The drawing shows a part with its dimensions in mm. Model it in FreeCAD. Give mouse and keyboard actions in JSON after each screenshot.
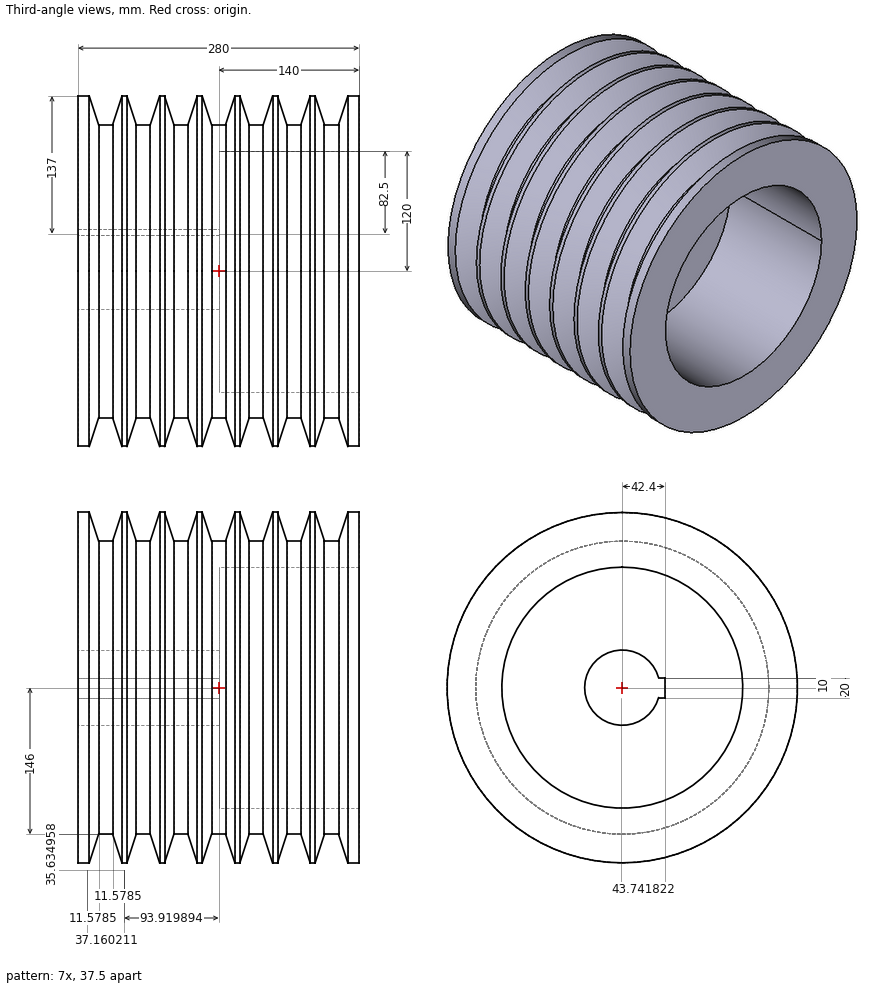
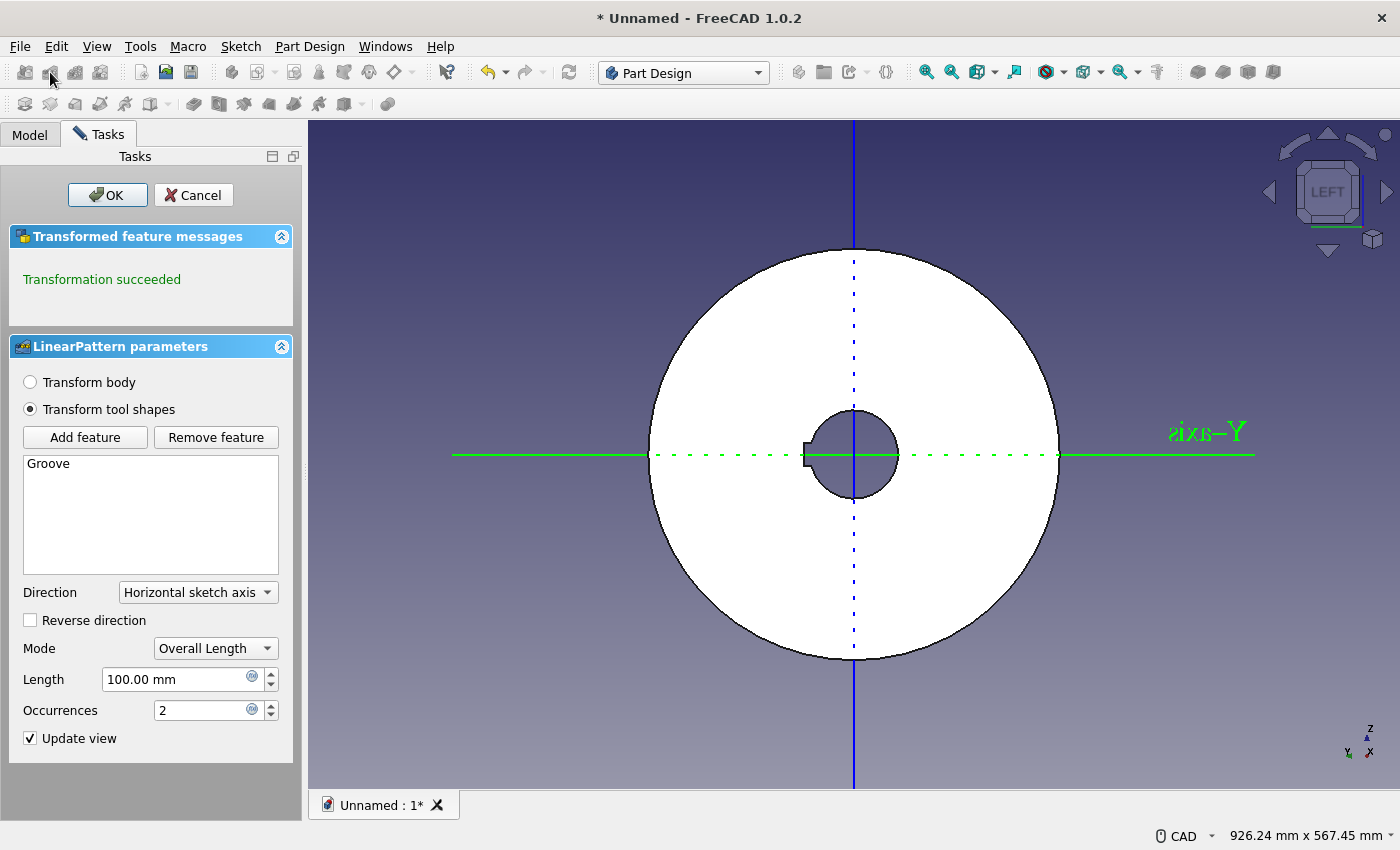
{"action": "left_click", "coordinate": [199, 592]}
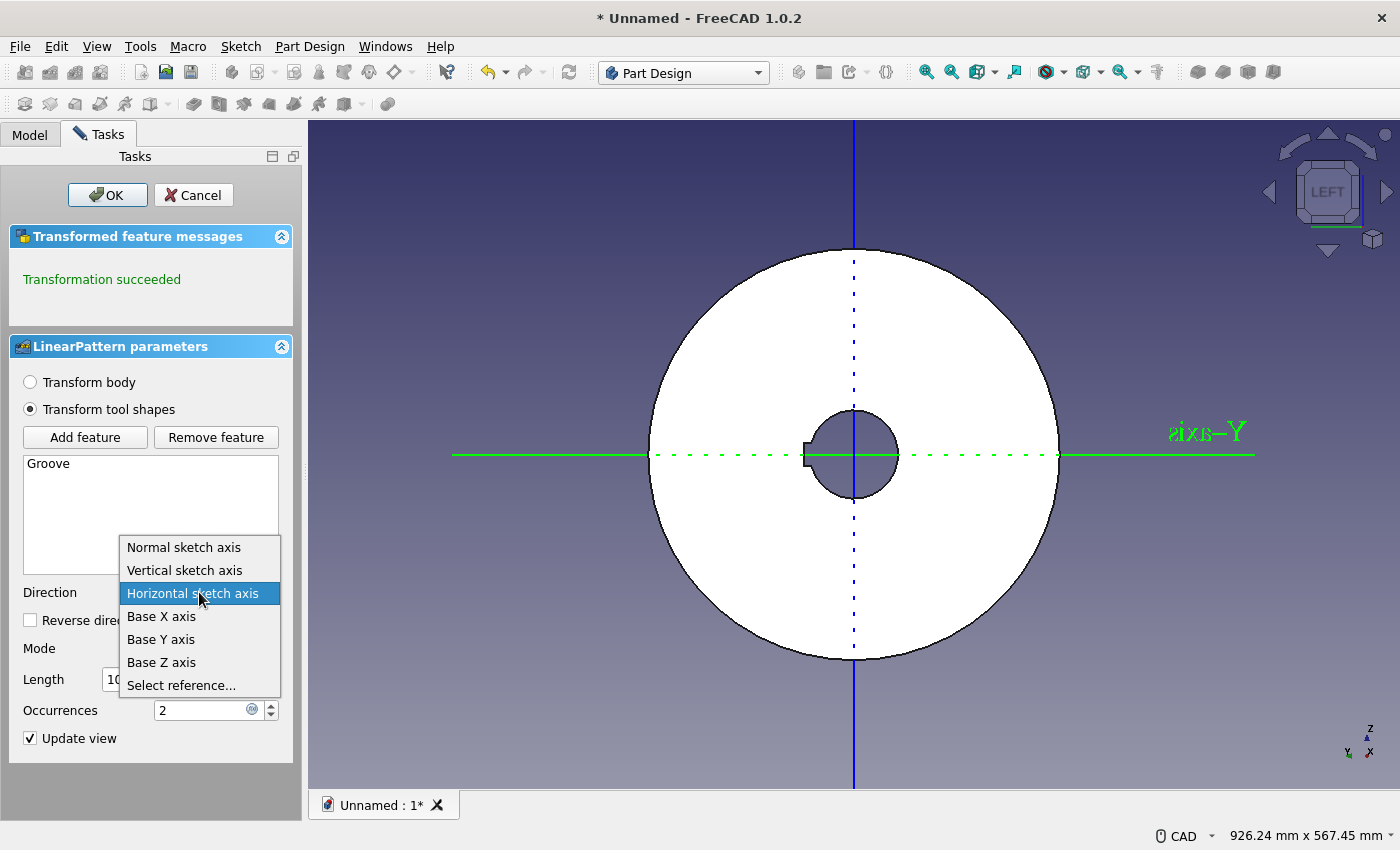
{"action": "left_click", "coordinate": [198, 616]}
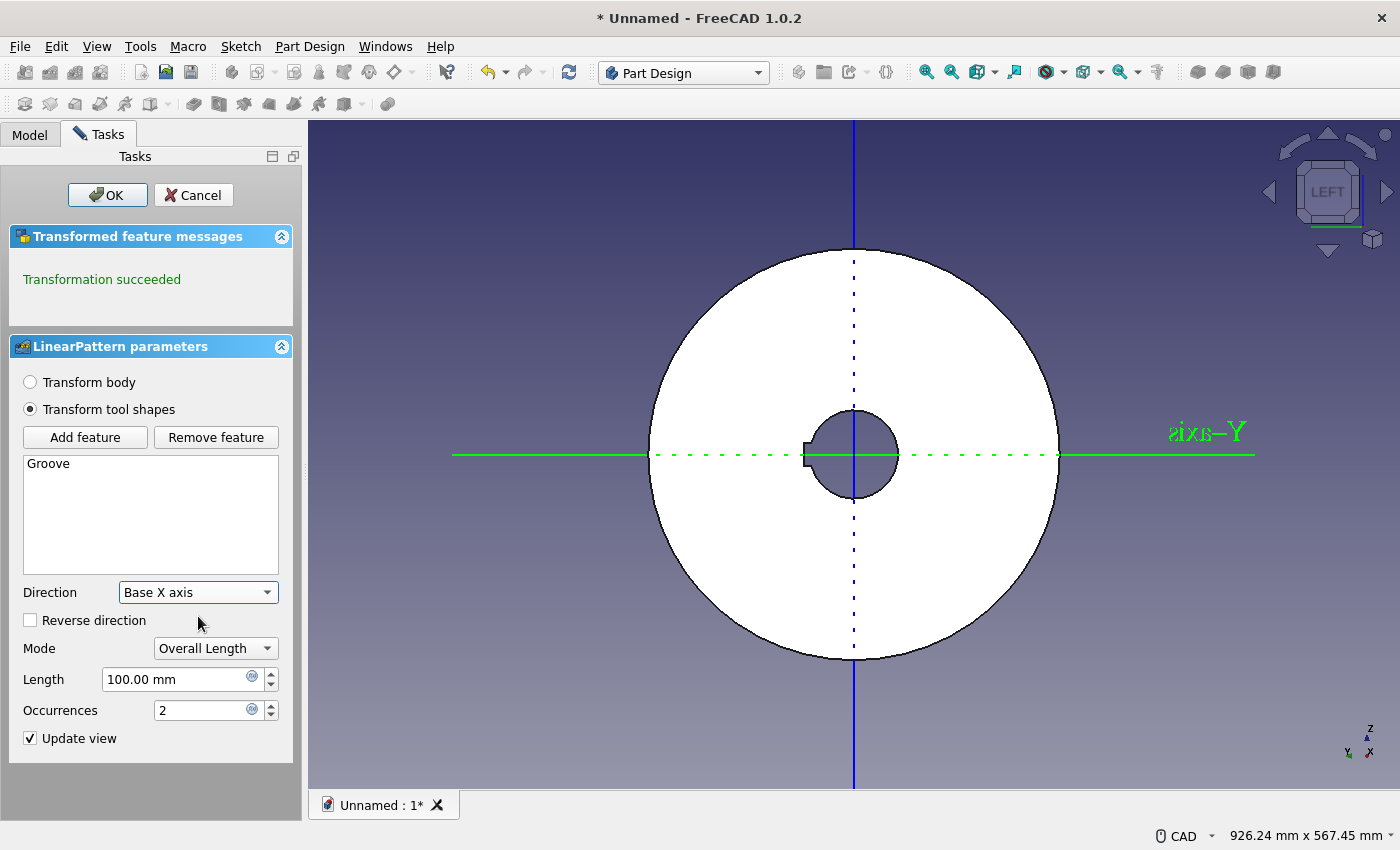
{"action": "left_click", "coordinate": [216, 648]}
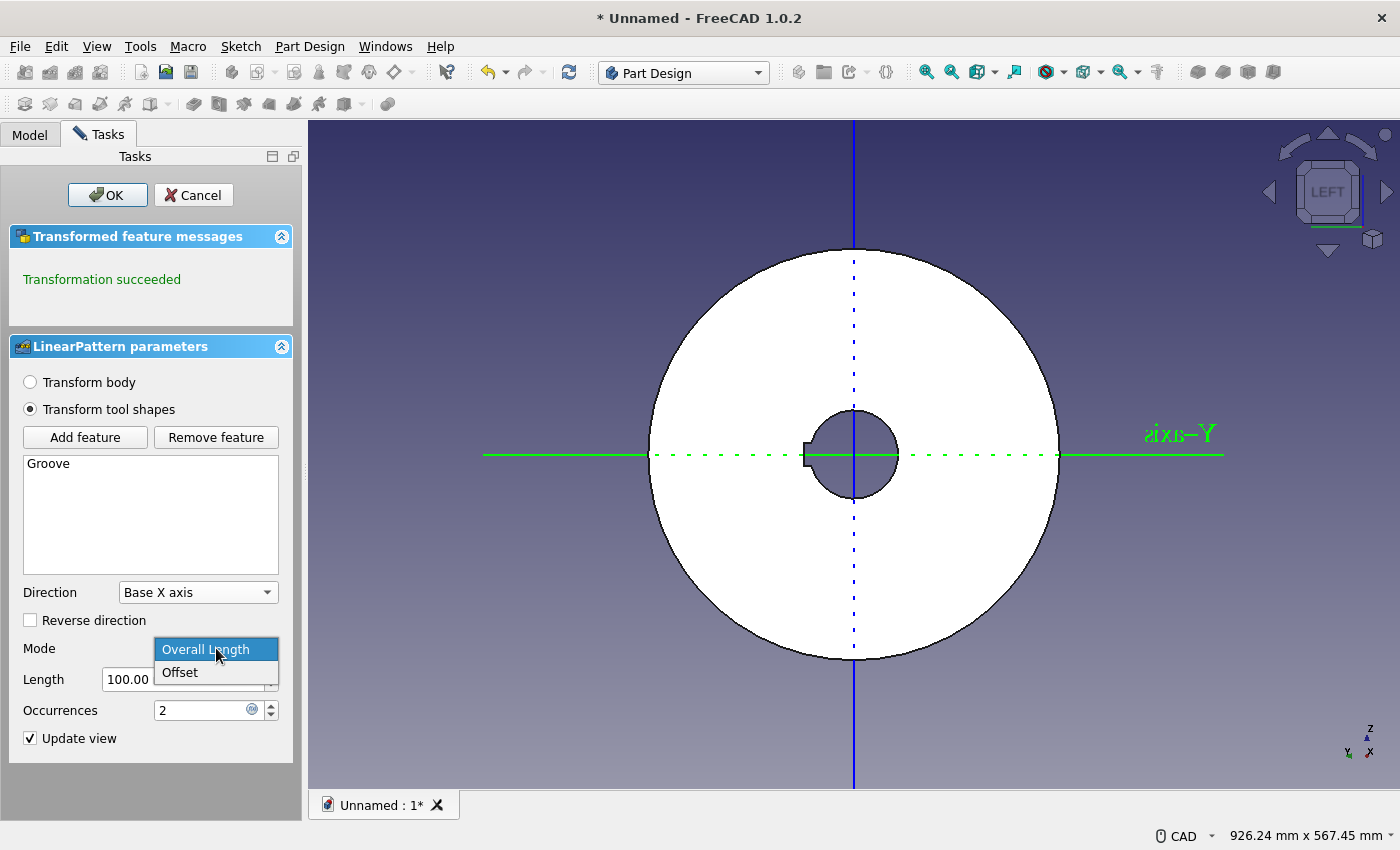
{"action": "left_click", "coordinate": [214, 672]}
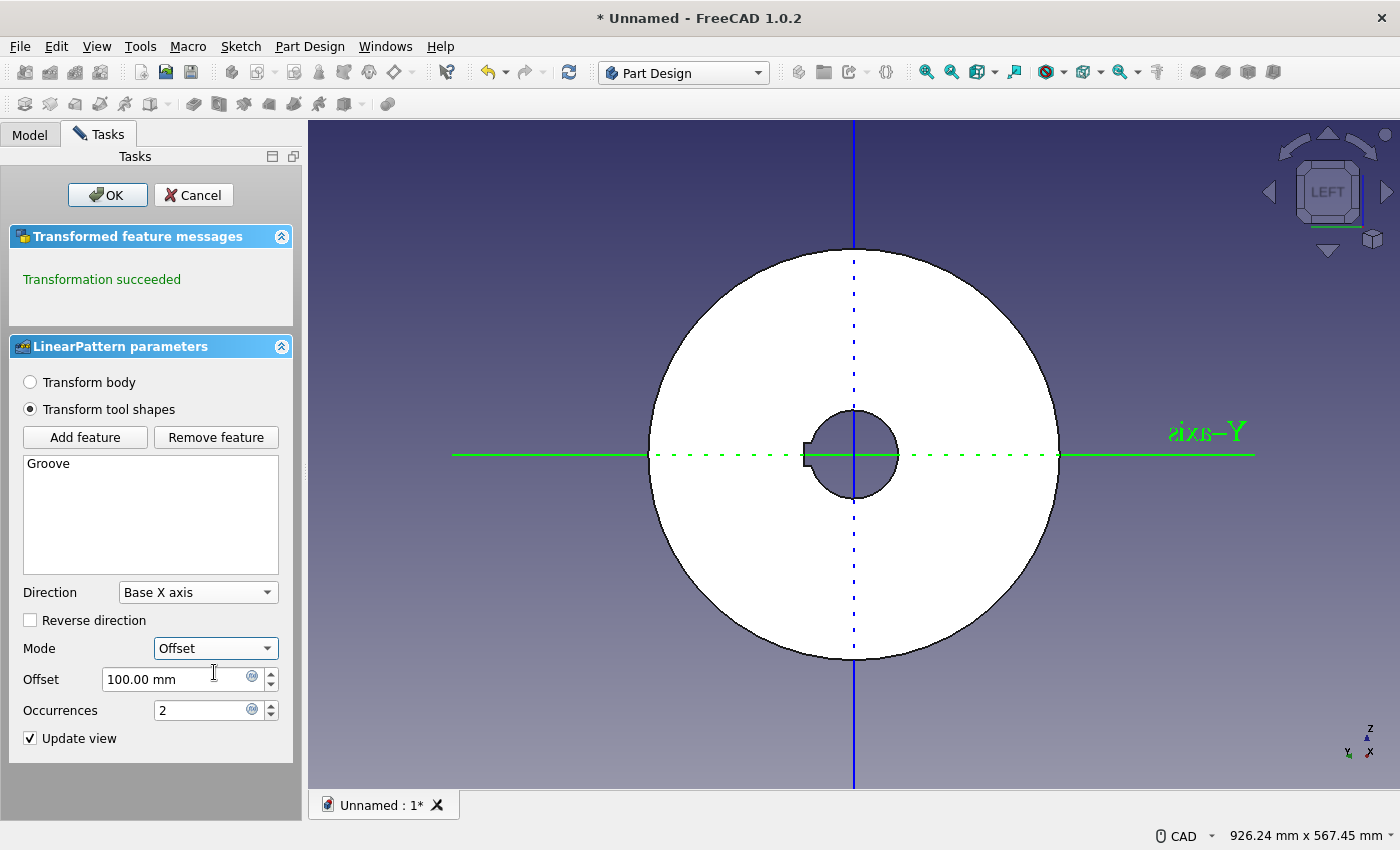
{"action": "triple_click", "coordinate": [184, 680]}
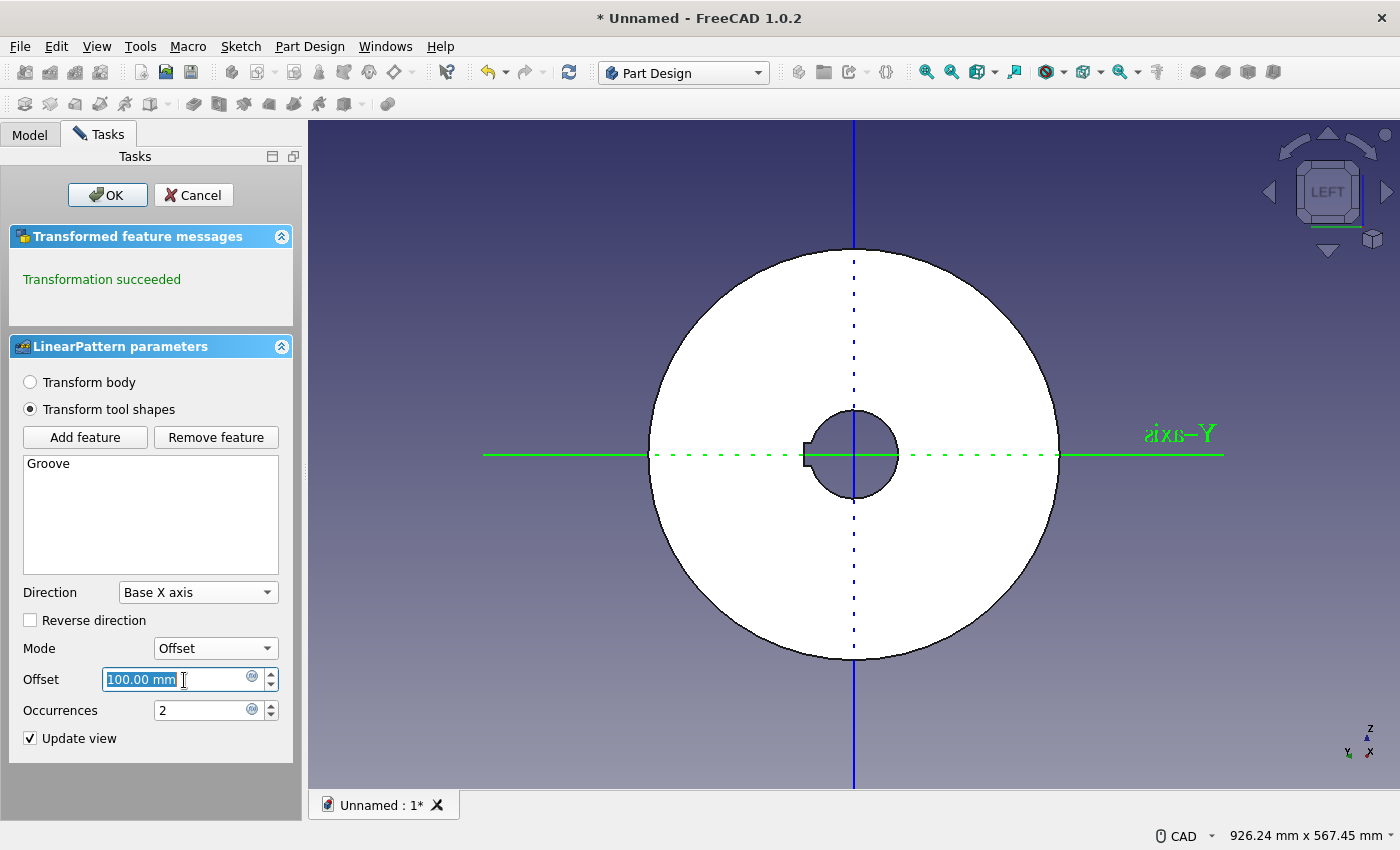
{"action": "type", "text": "37.5"}
{"action": "key", "text": "Tab"}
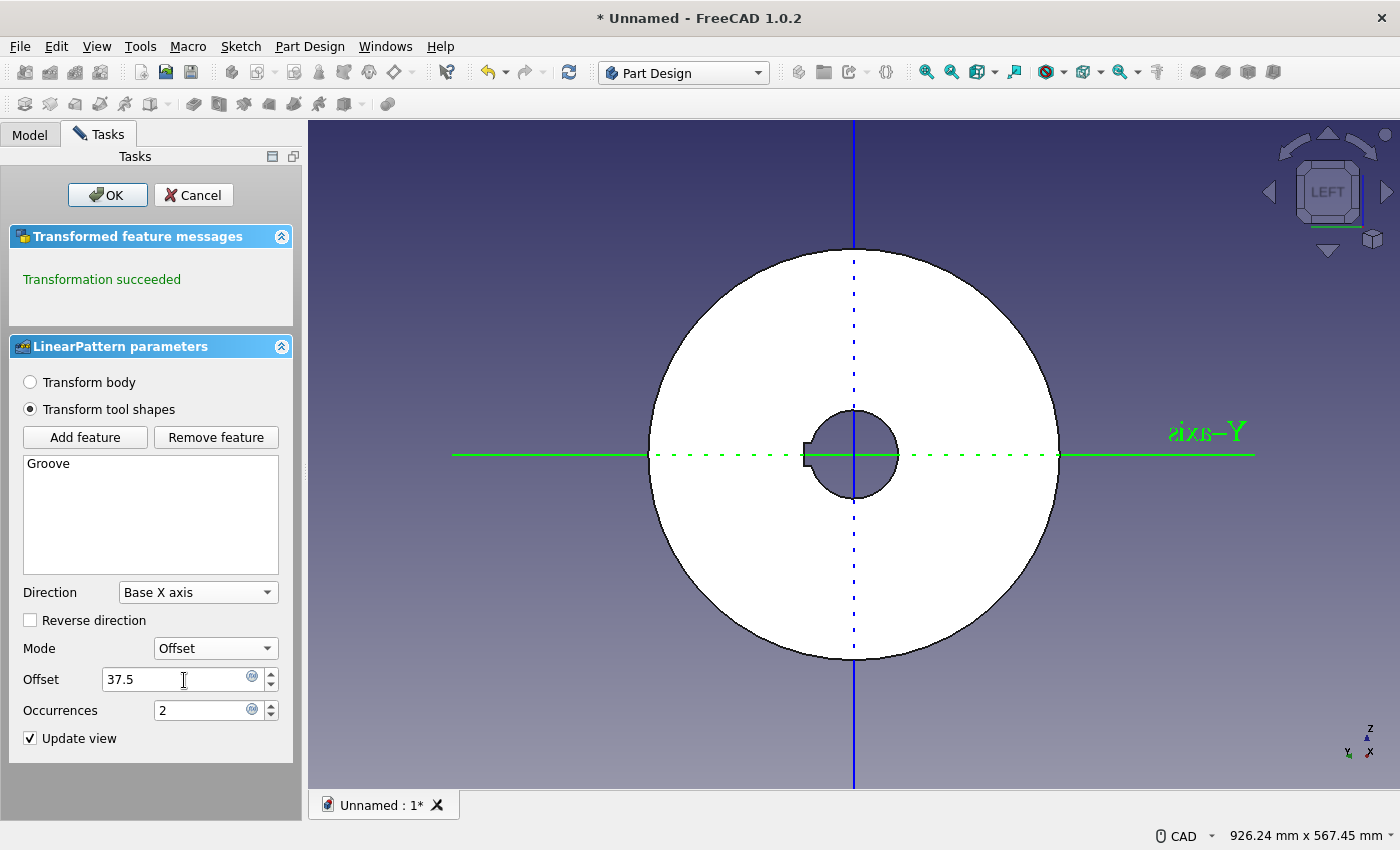
{"action": "triple_click", "coordinate": [210, 710]}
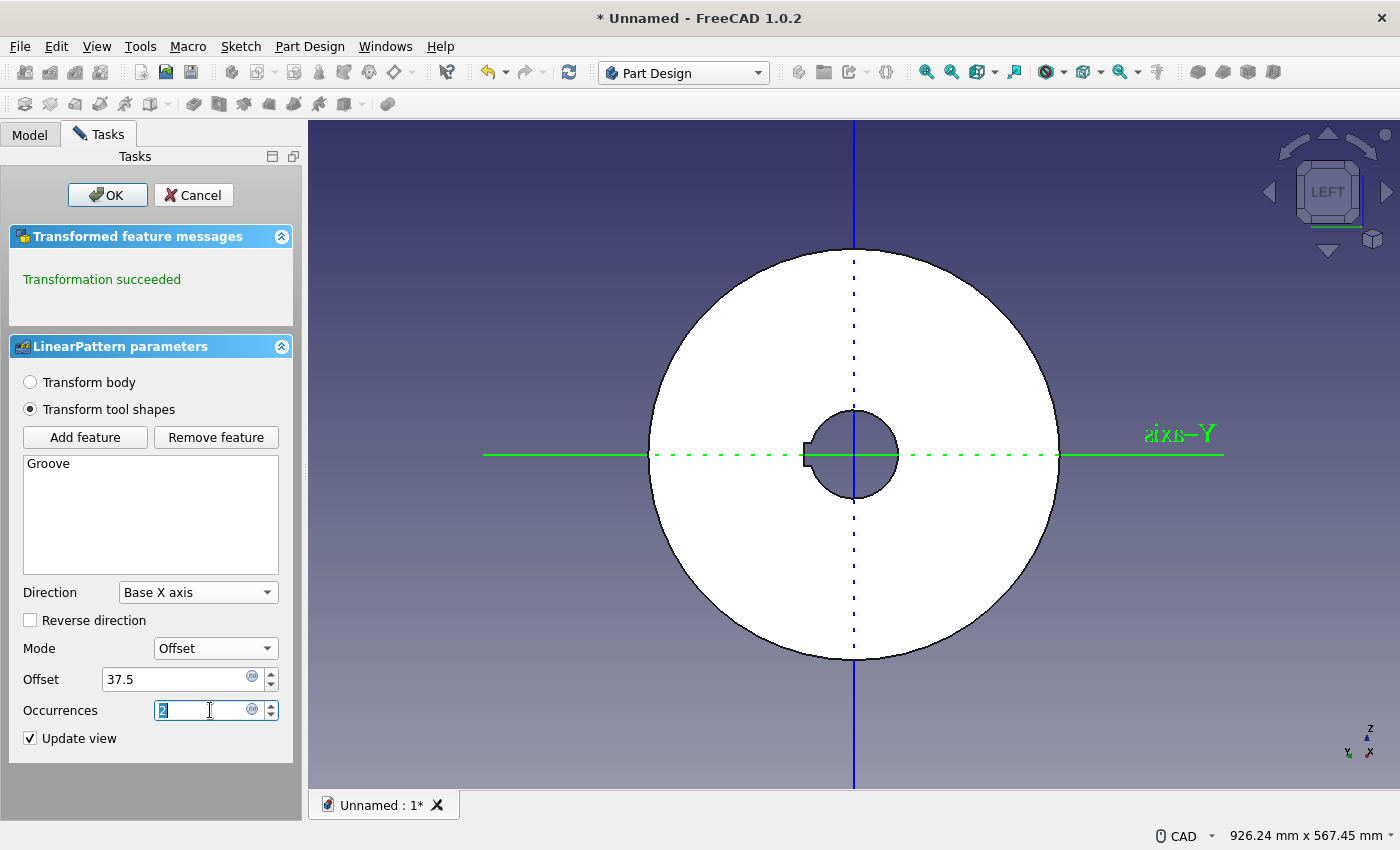
{"action": "type", "text": "7"}
{"action": "key", "text": "Tab"}